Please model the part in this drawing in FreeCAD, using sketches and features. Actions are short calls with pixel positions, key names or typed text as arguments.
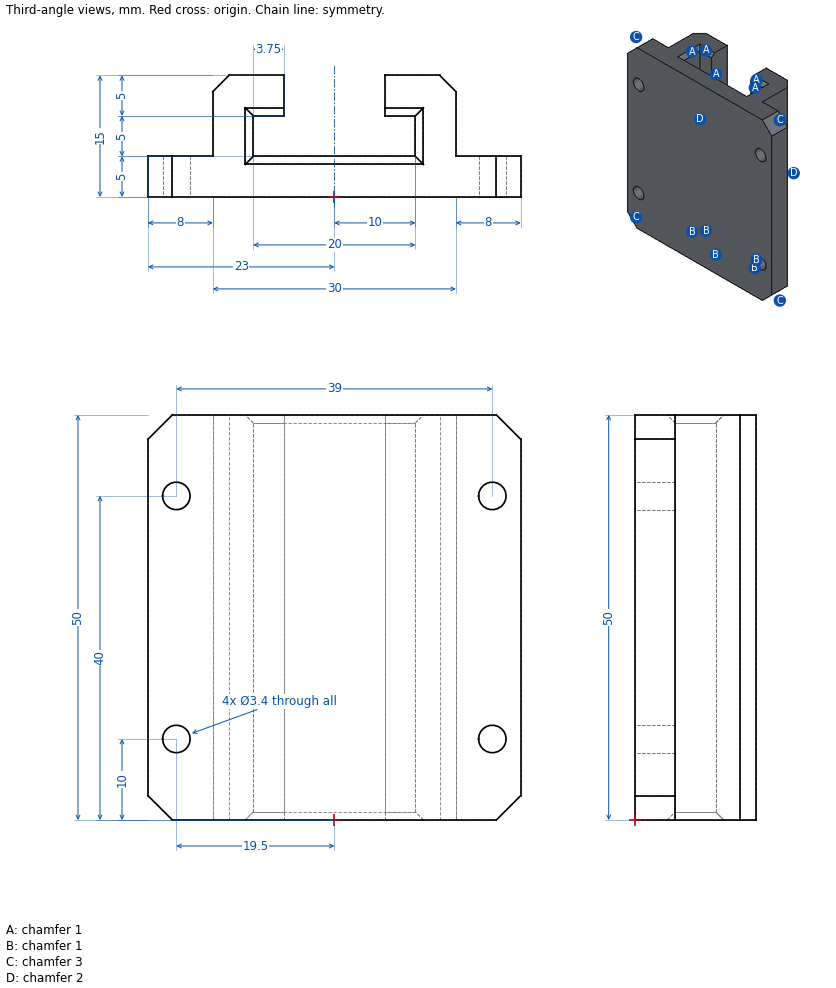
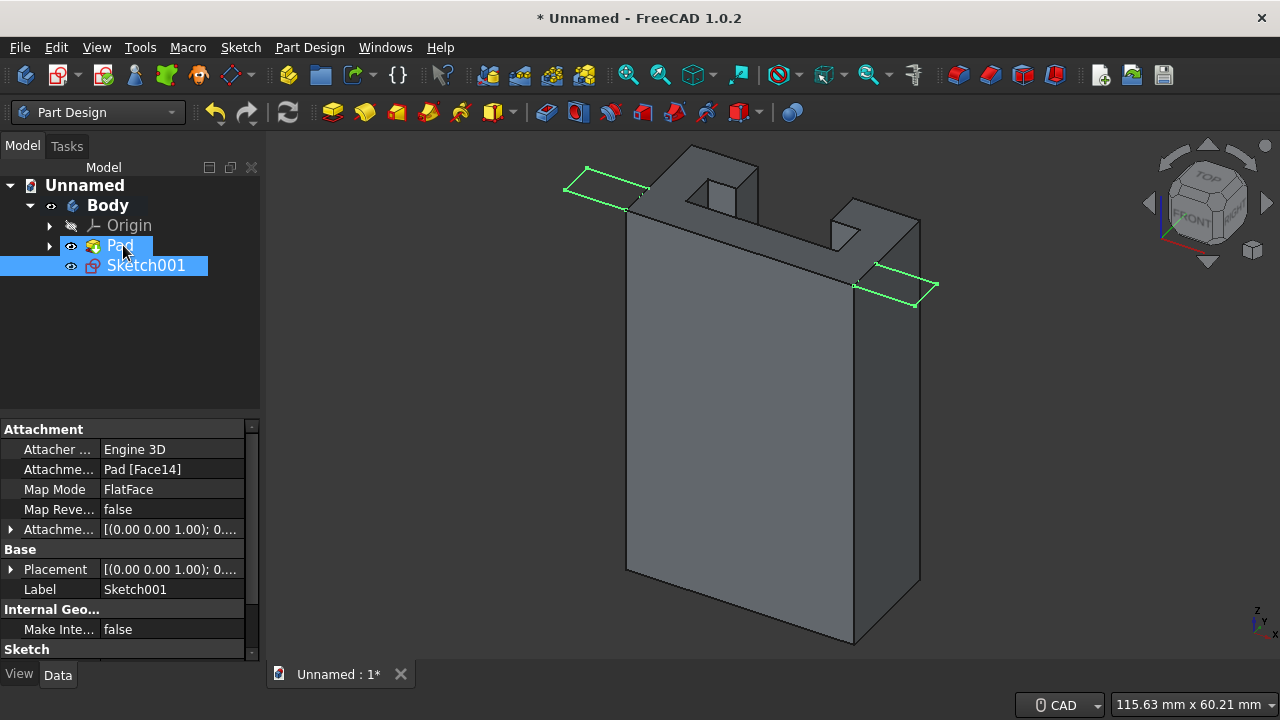
click(334, 112)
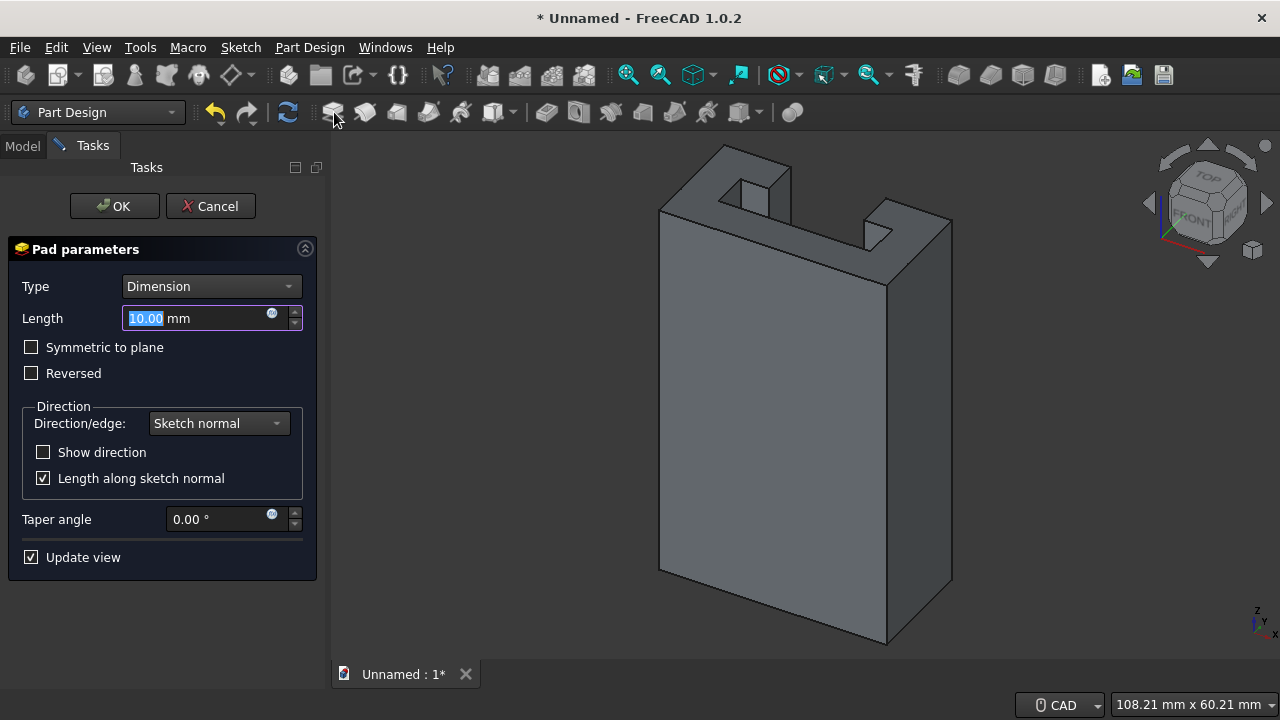
text(50)
key(Tab)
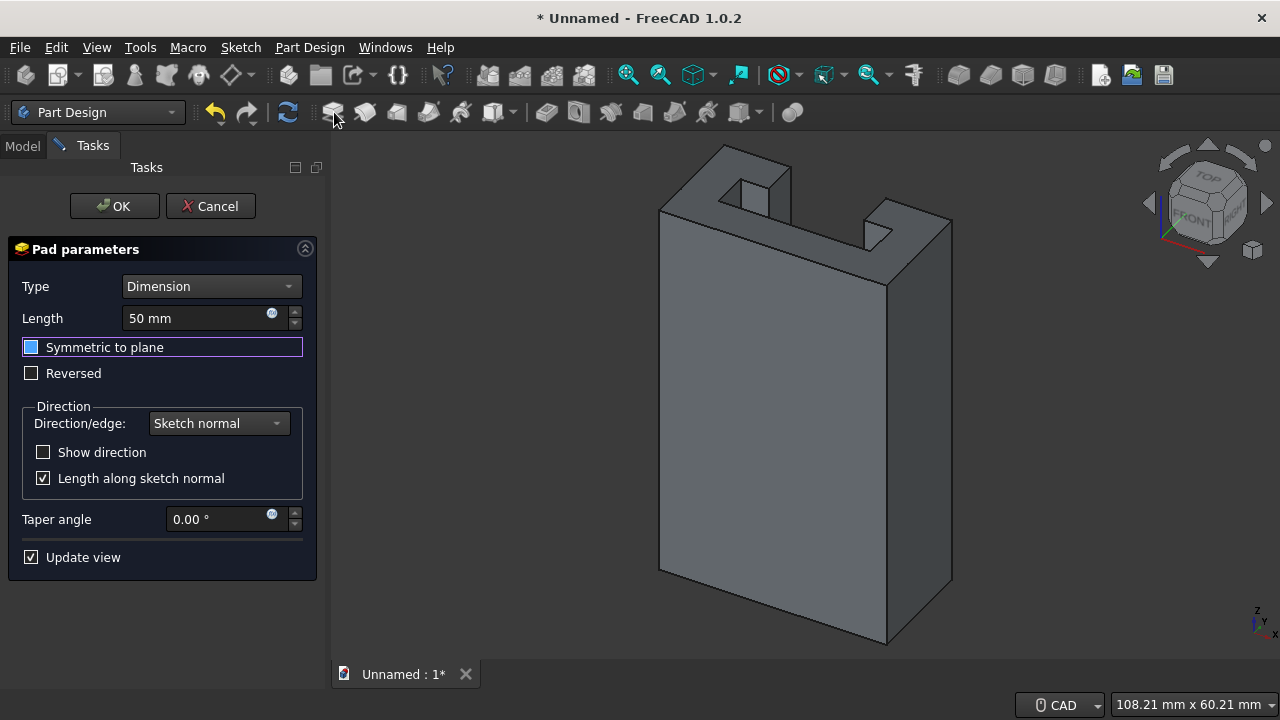
click(30, 373)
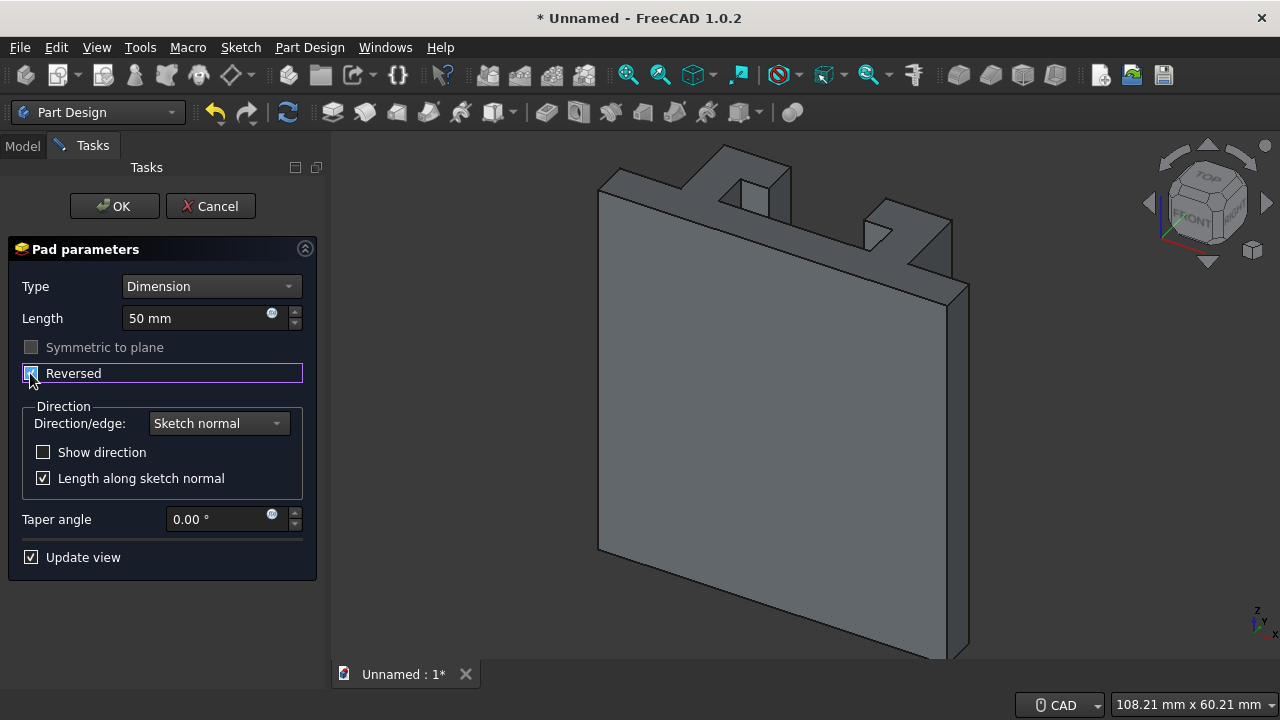
click(115, 206)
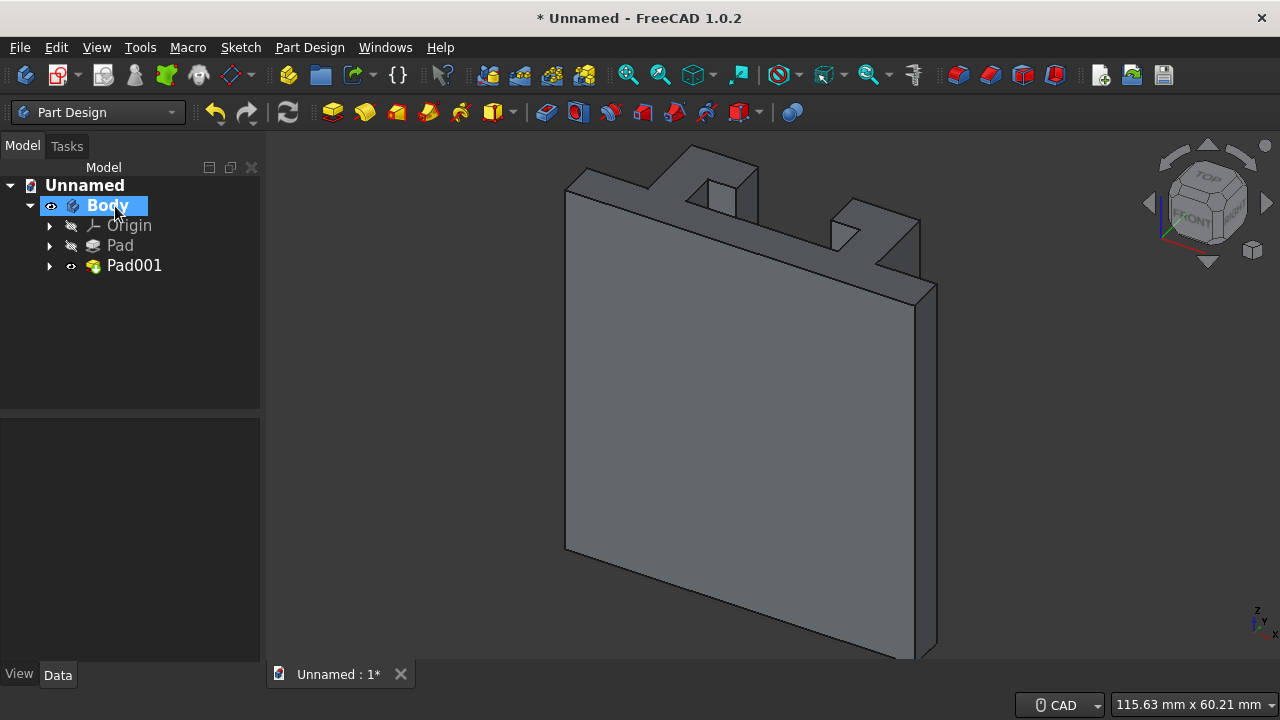
click(630, 76)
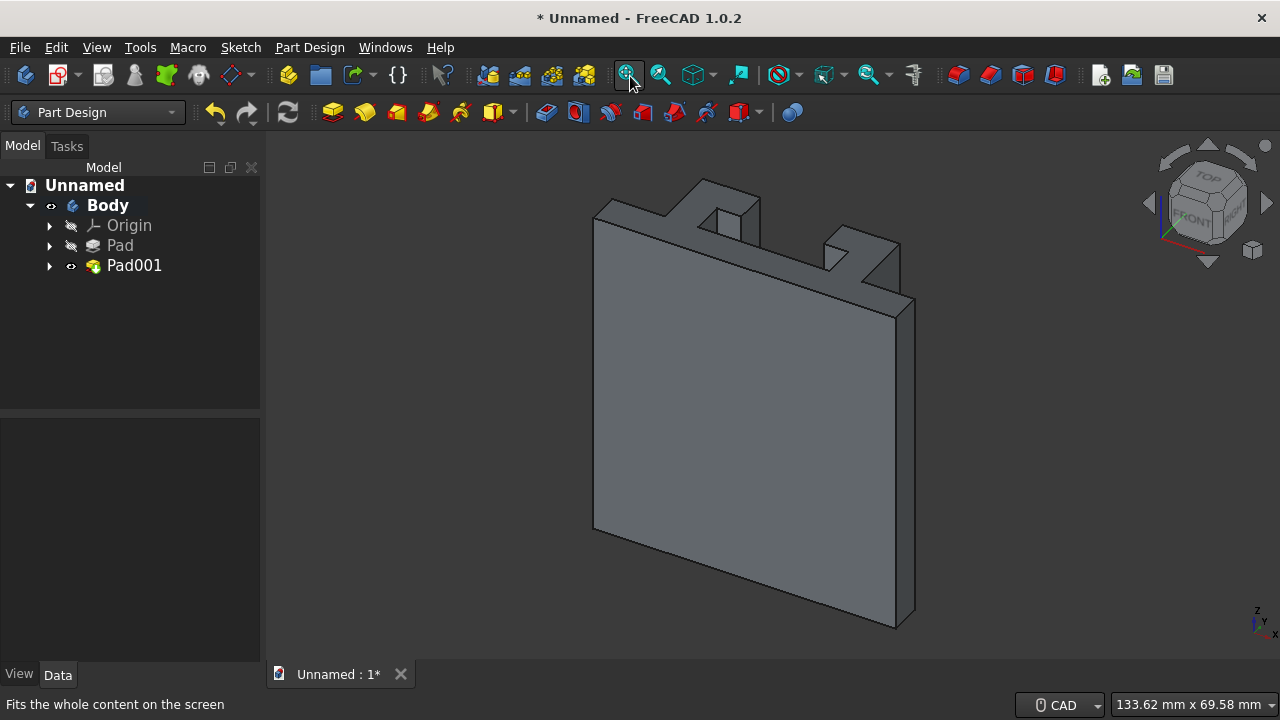
click(836, 247)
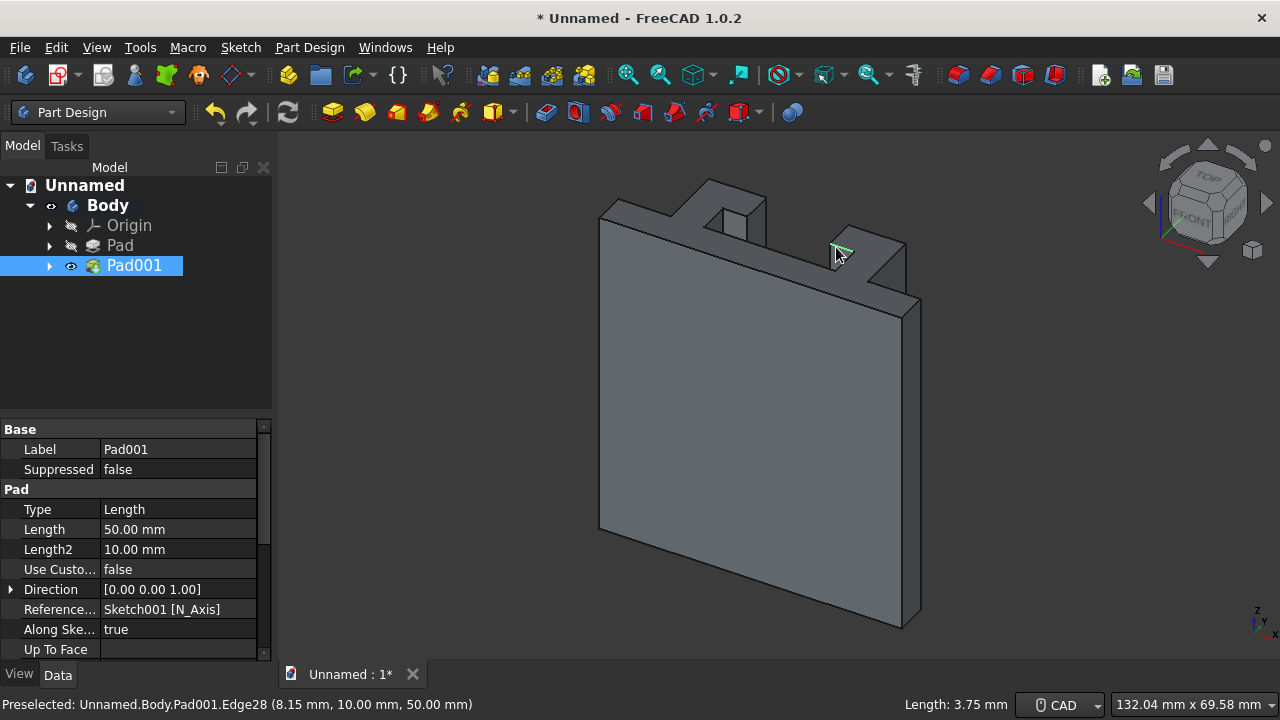
click(713, 217, ctrl)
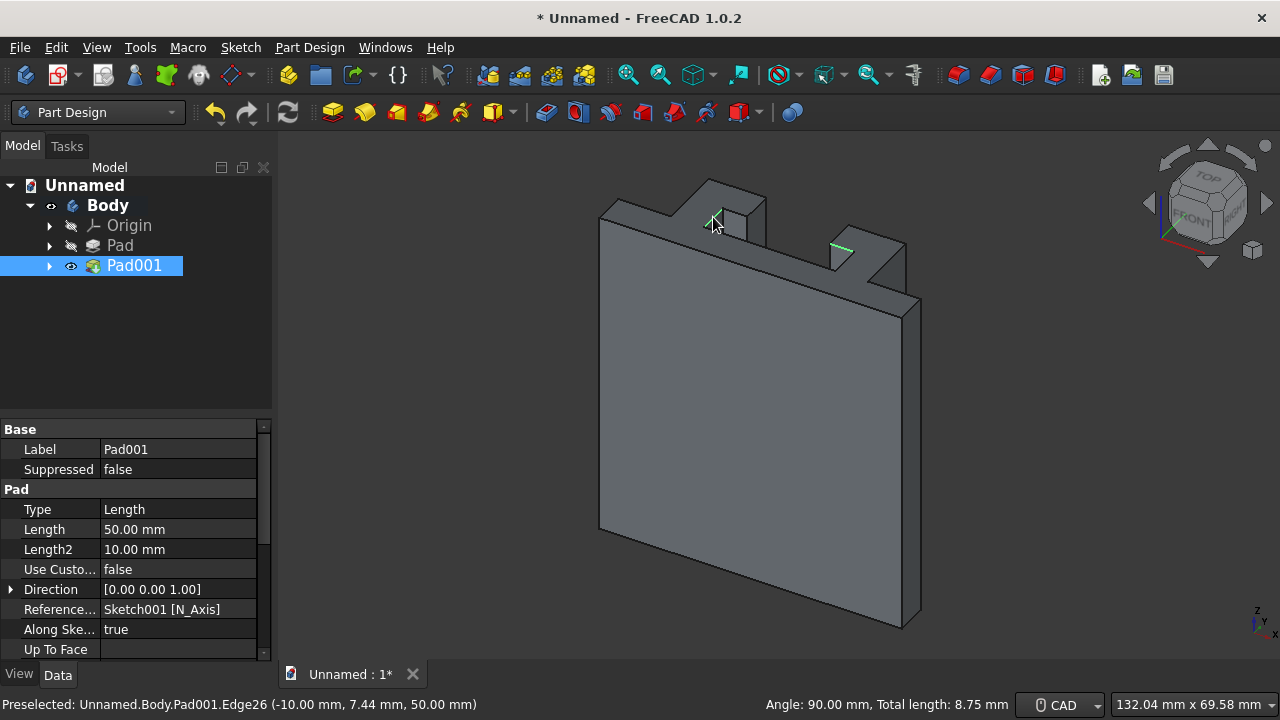
click(735, 211, ctrl)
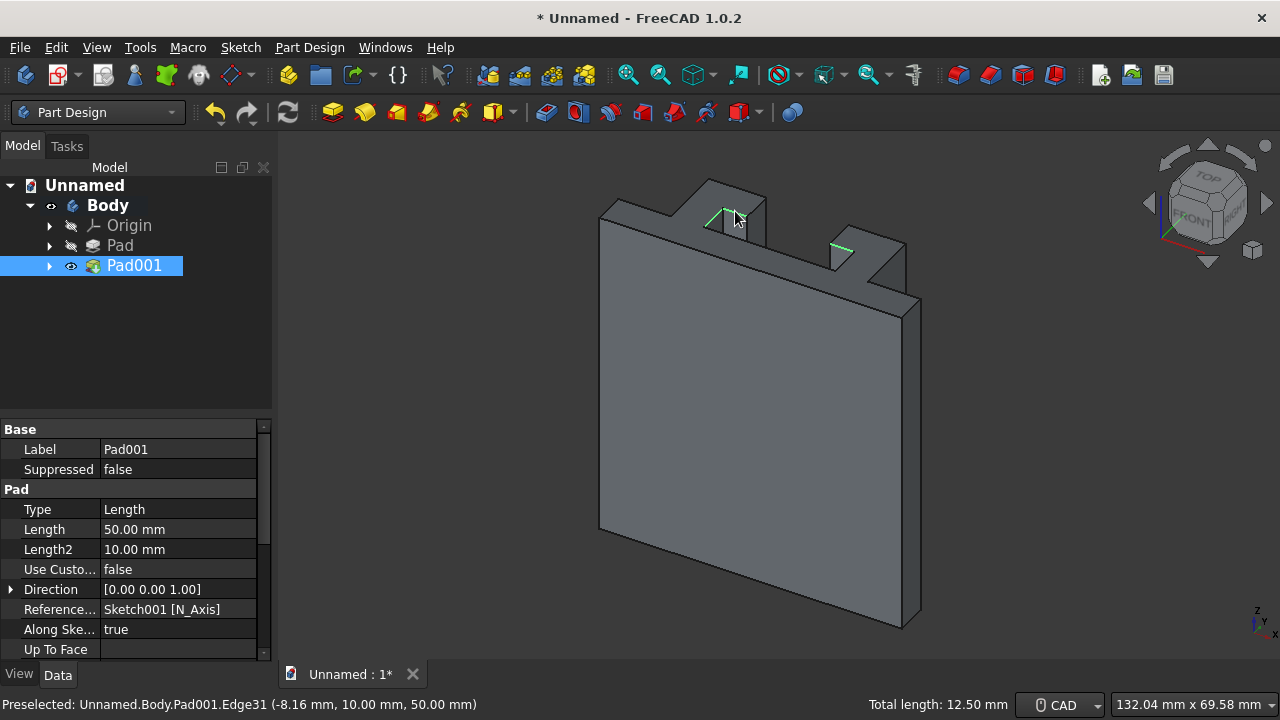
key(0)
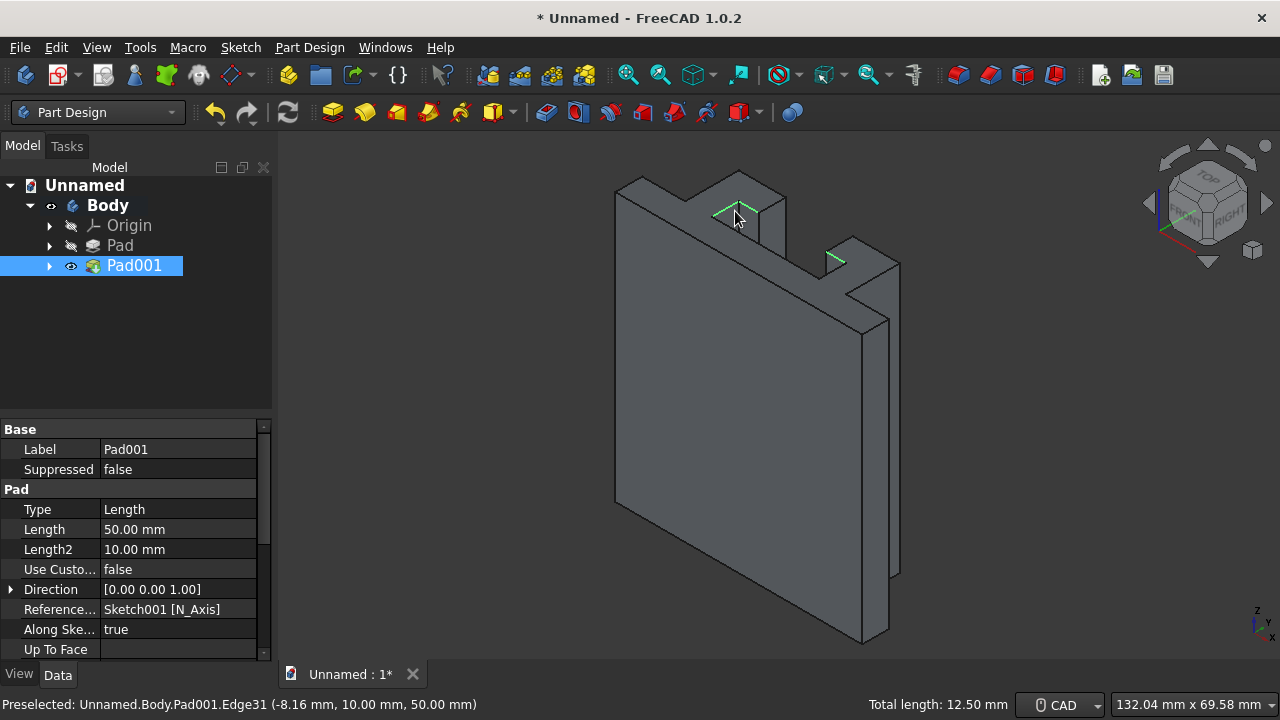
key(2)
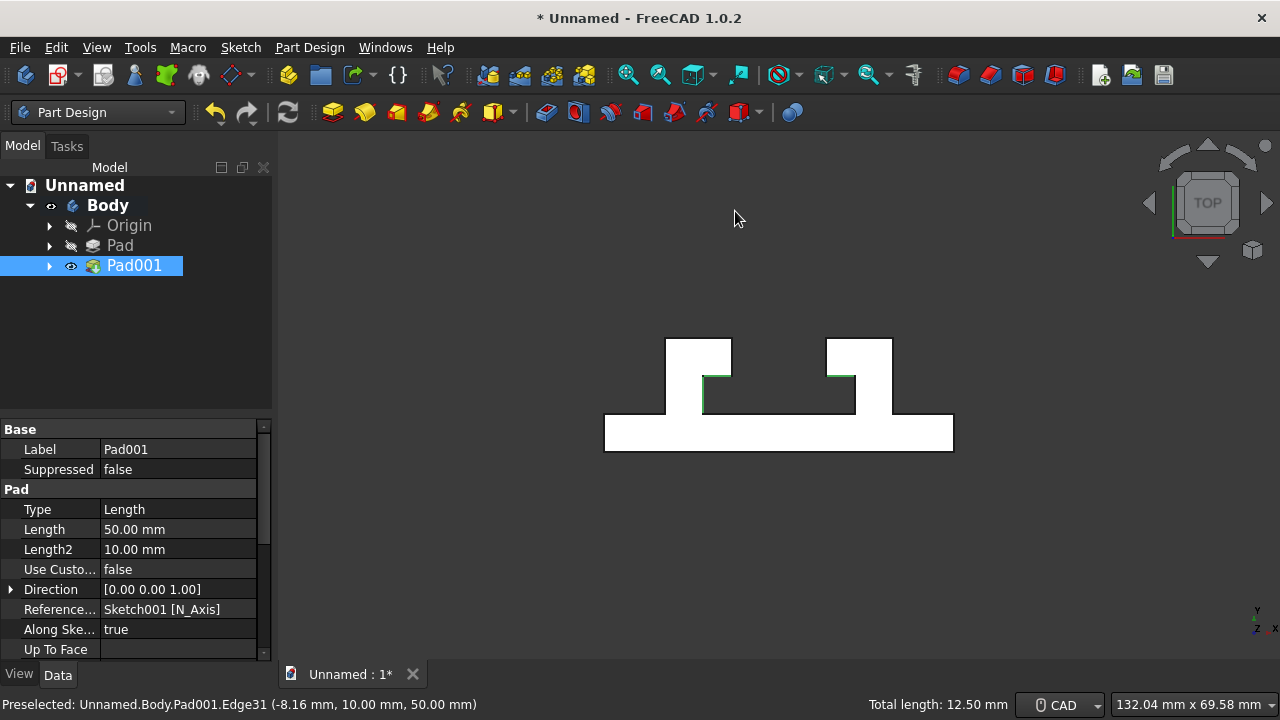
key(v)
key(f)